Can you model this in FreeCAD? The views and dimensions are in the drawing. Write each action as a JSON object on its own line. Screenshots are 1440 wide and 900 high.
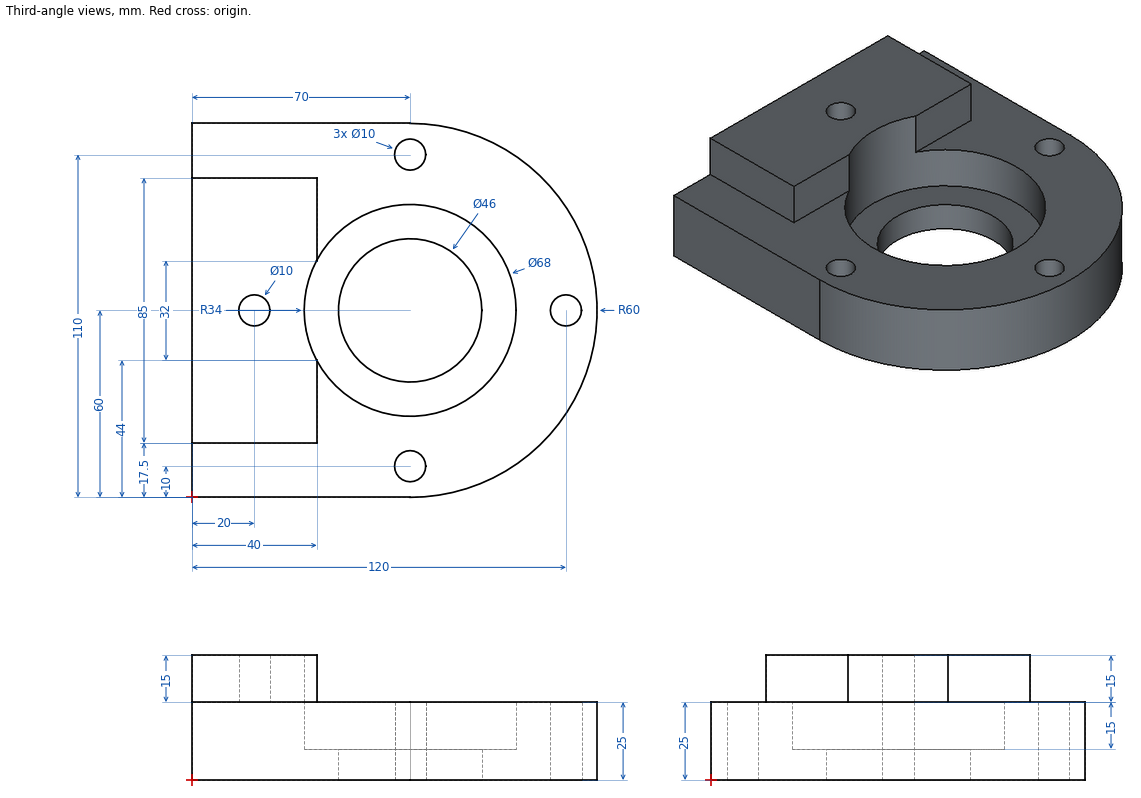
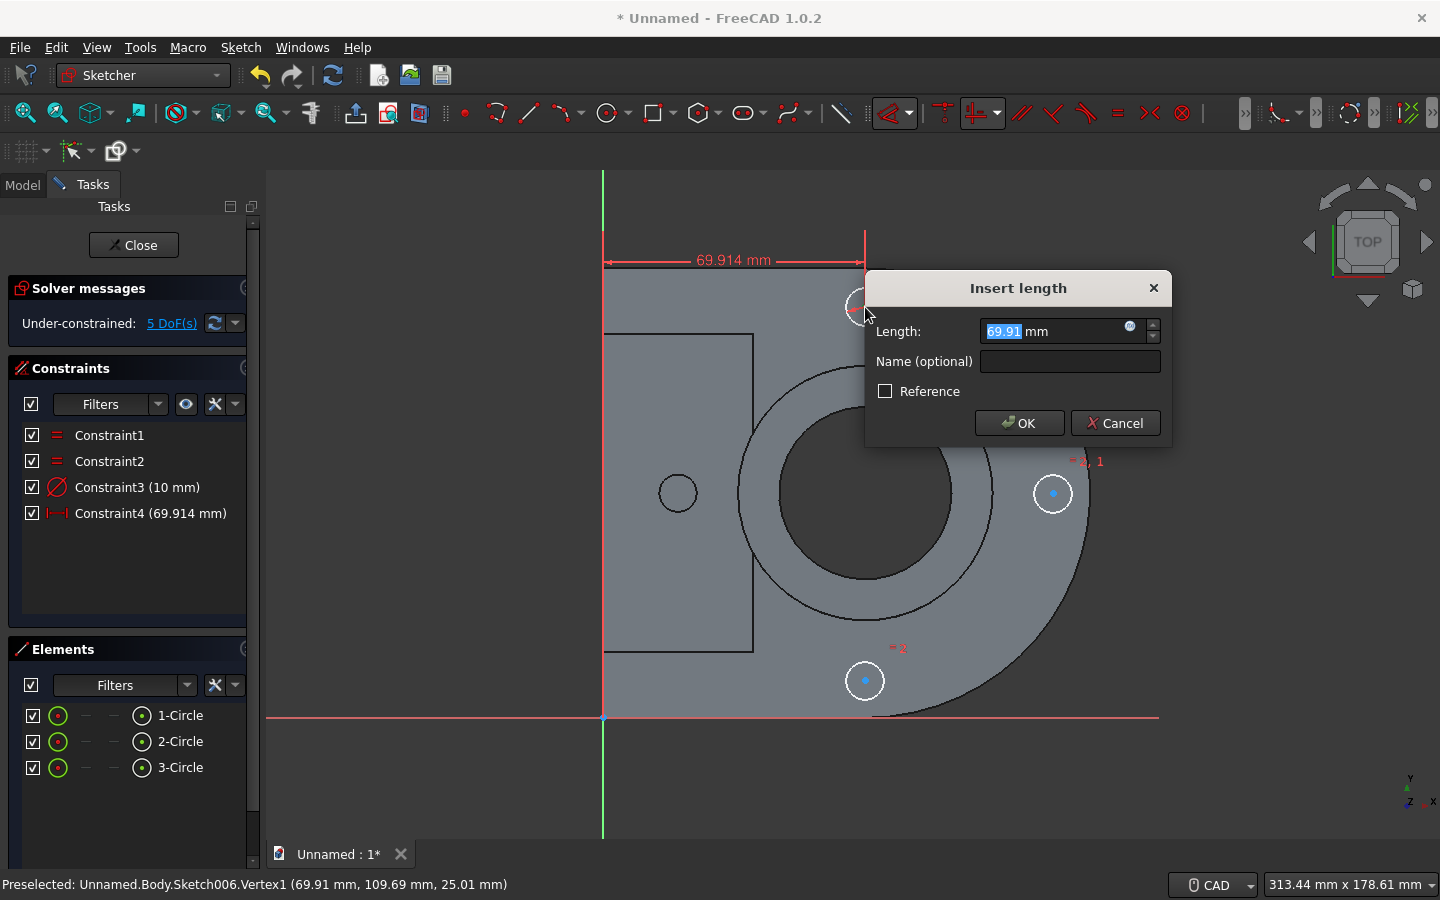
{"action": "type", "text": "70"}
{"action": "key", "text": "Return"}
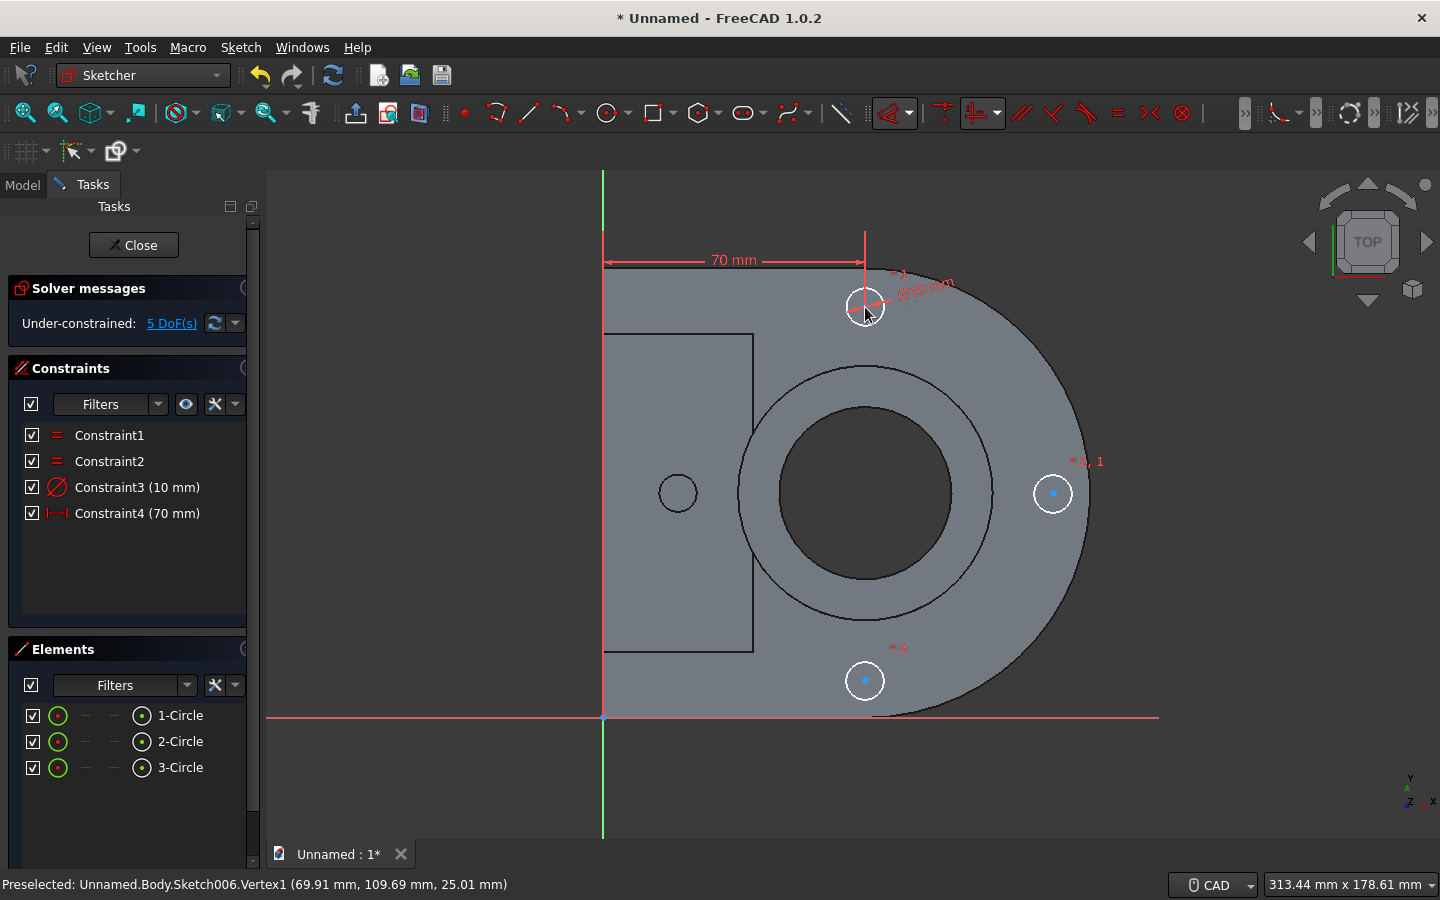
{"action": "left_click", "coordinate": [1053, 494]}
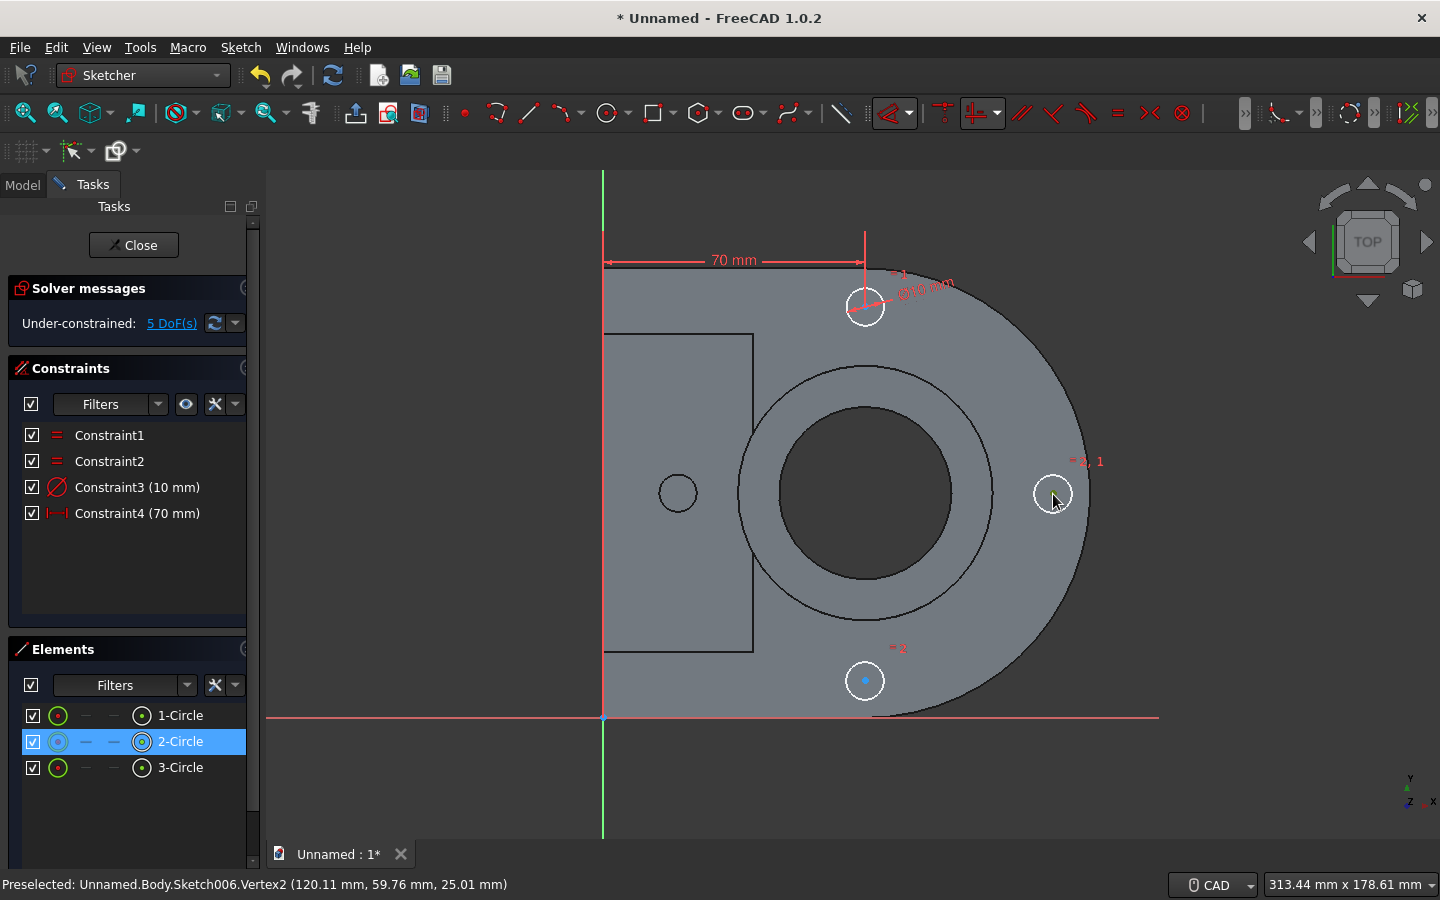
{"action": "left_click", "coordinate": [912, 114]}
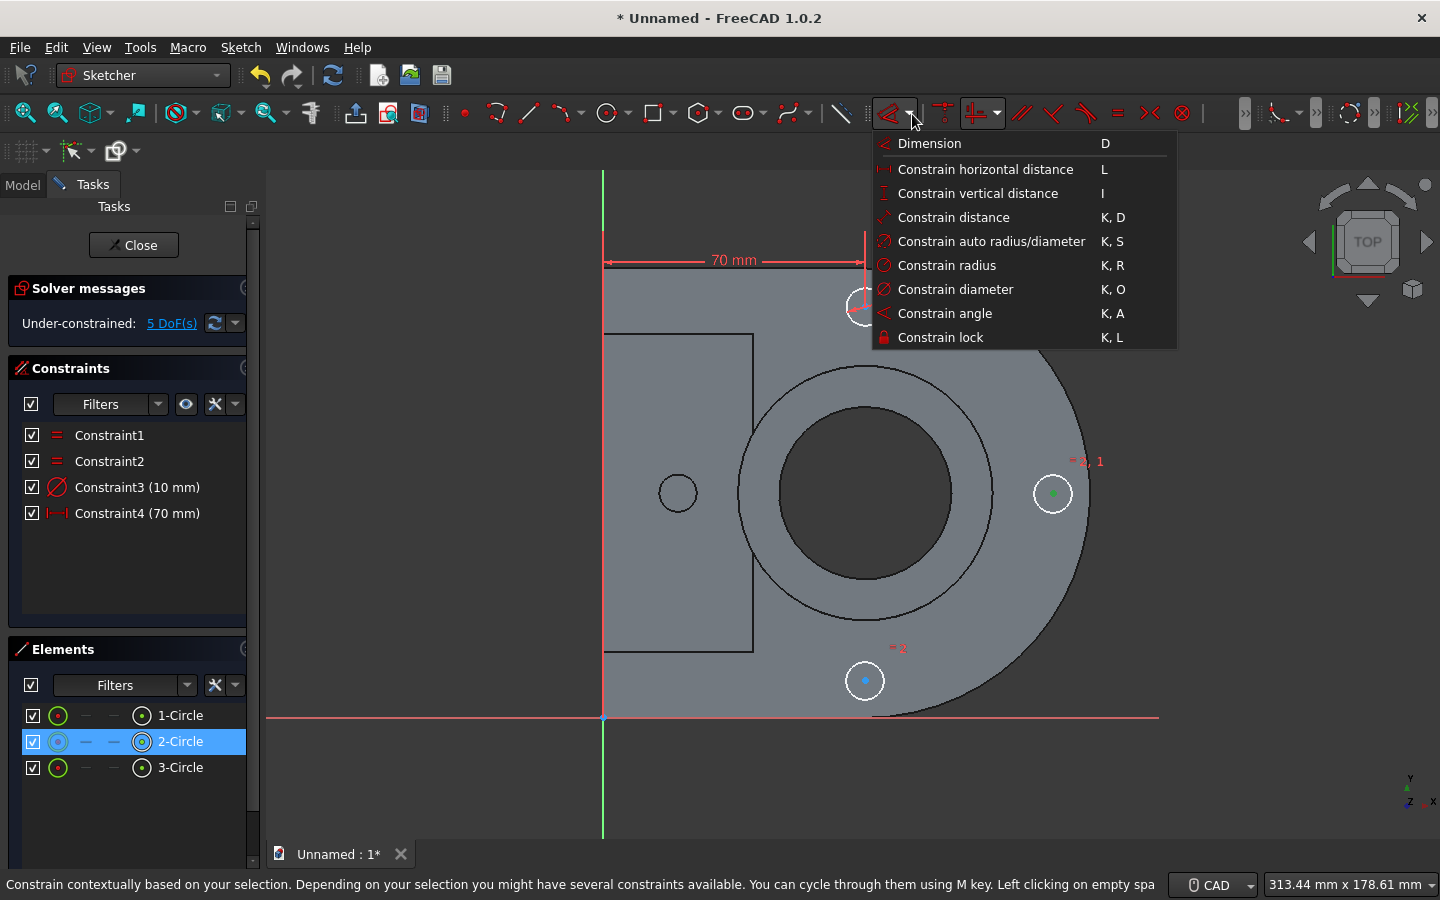
{"action": "left_click", "coordinate": [1025, 193]}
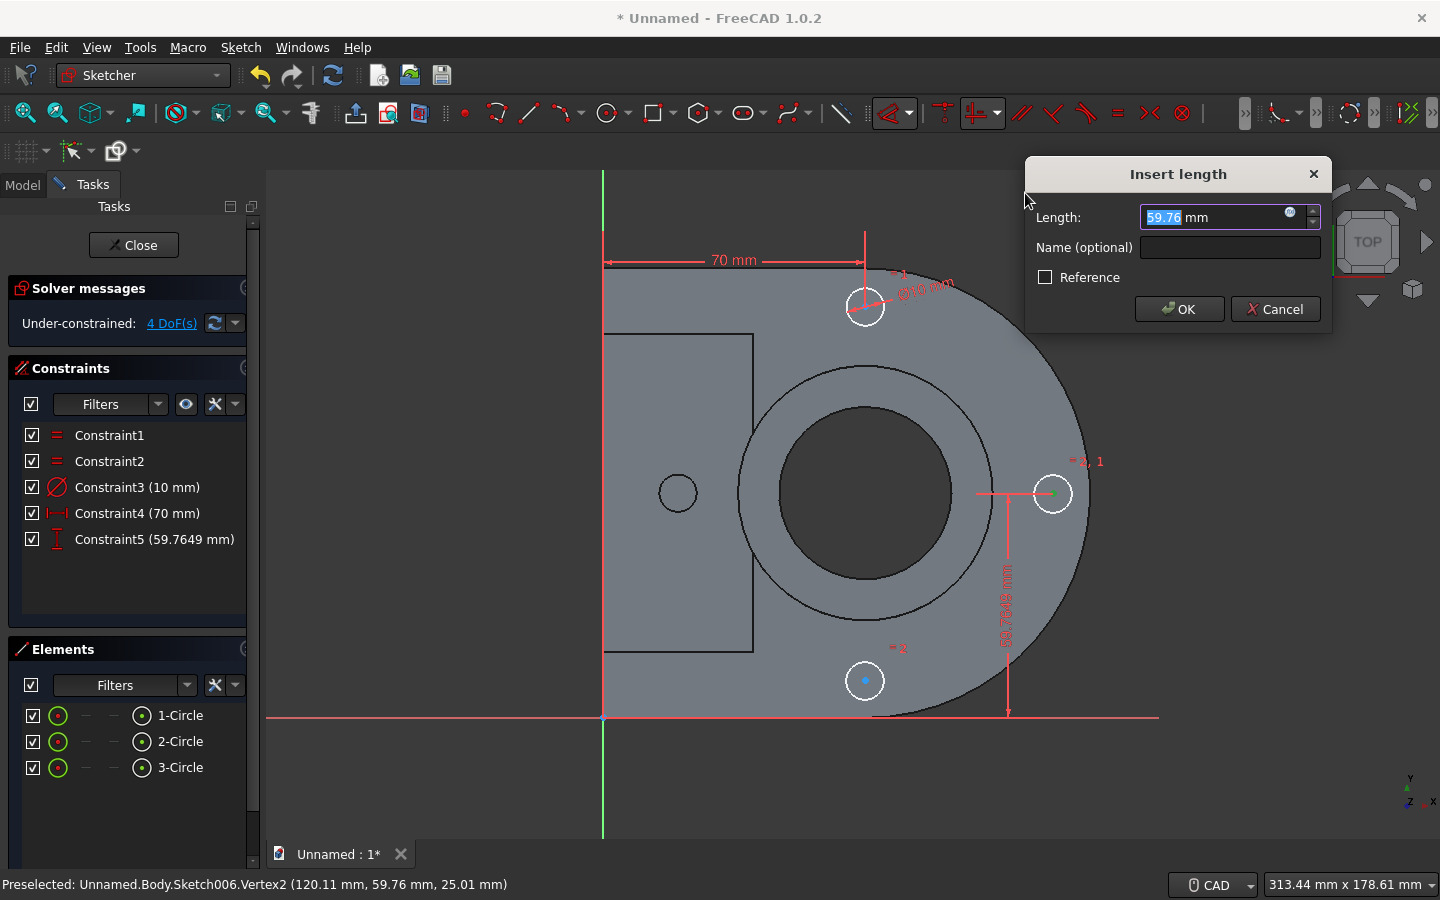
{"action": "type", "text": "60"}
{"action": "key", "text": "Return"}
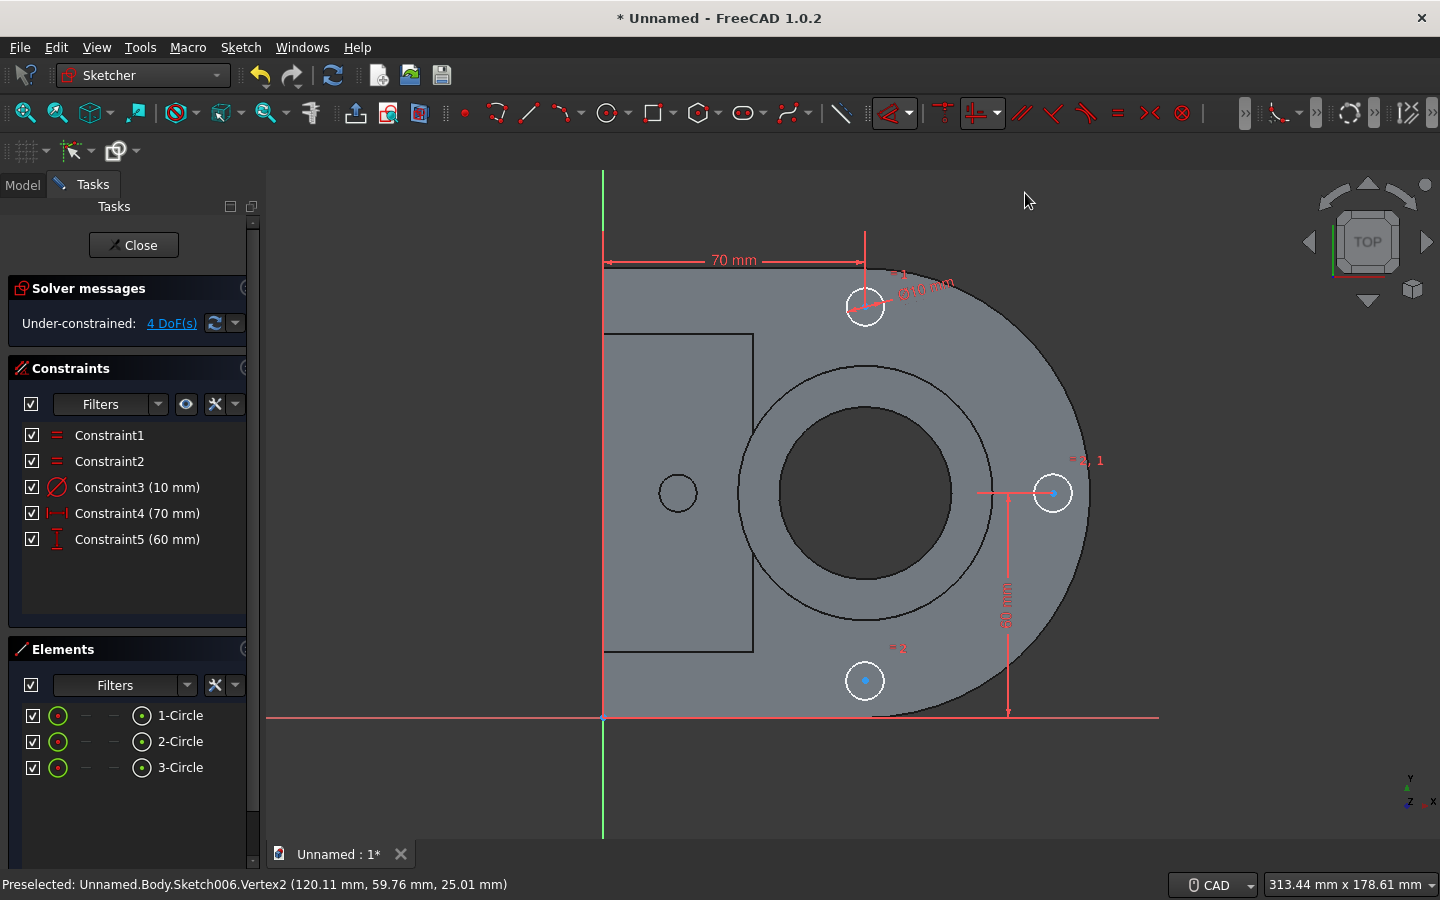
{"action": "left_click", "coordinate": [865, 681]}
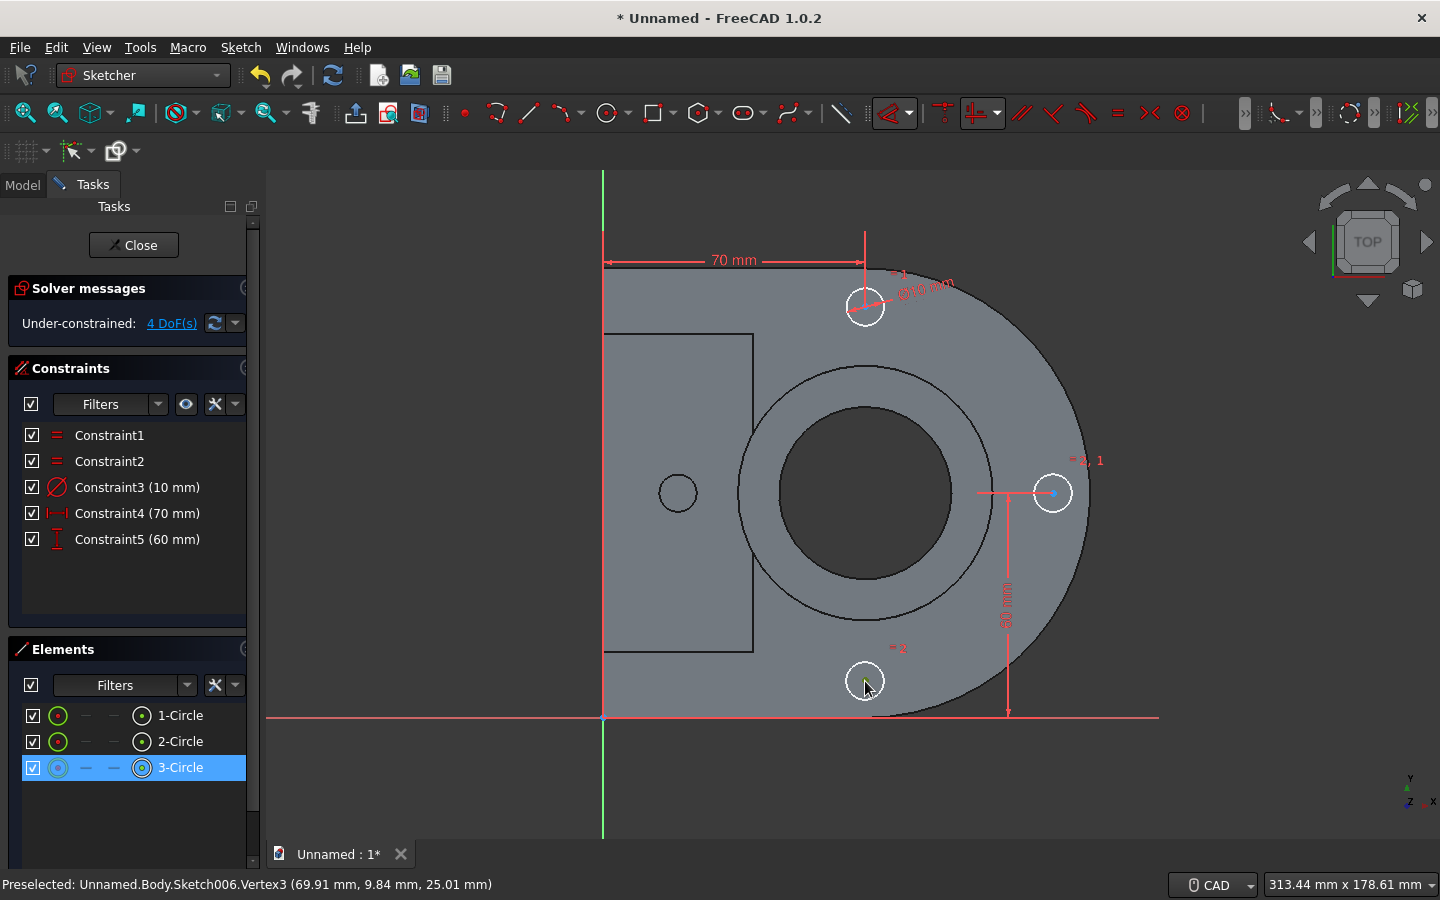
{"action": "left_click", "coordinate": [912, 114]}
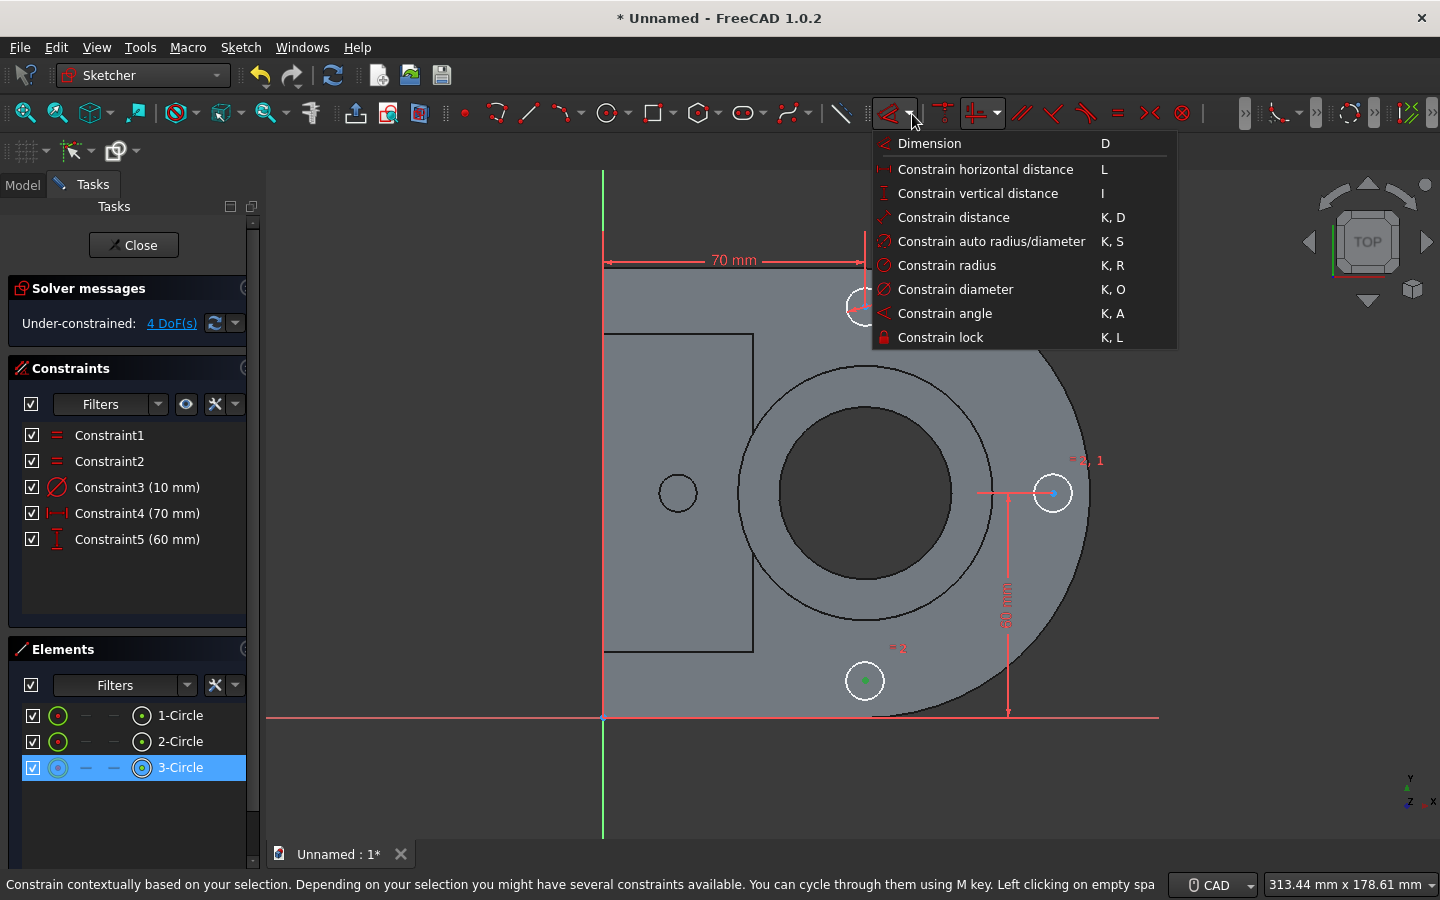
{"action": "left_click", "coordinate": [1025, 169]}